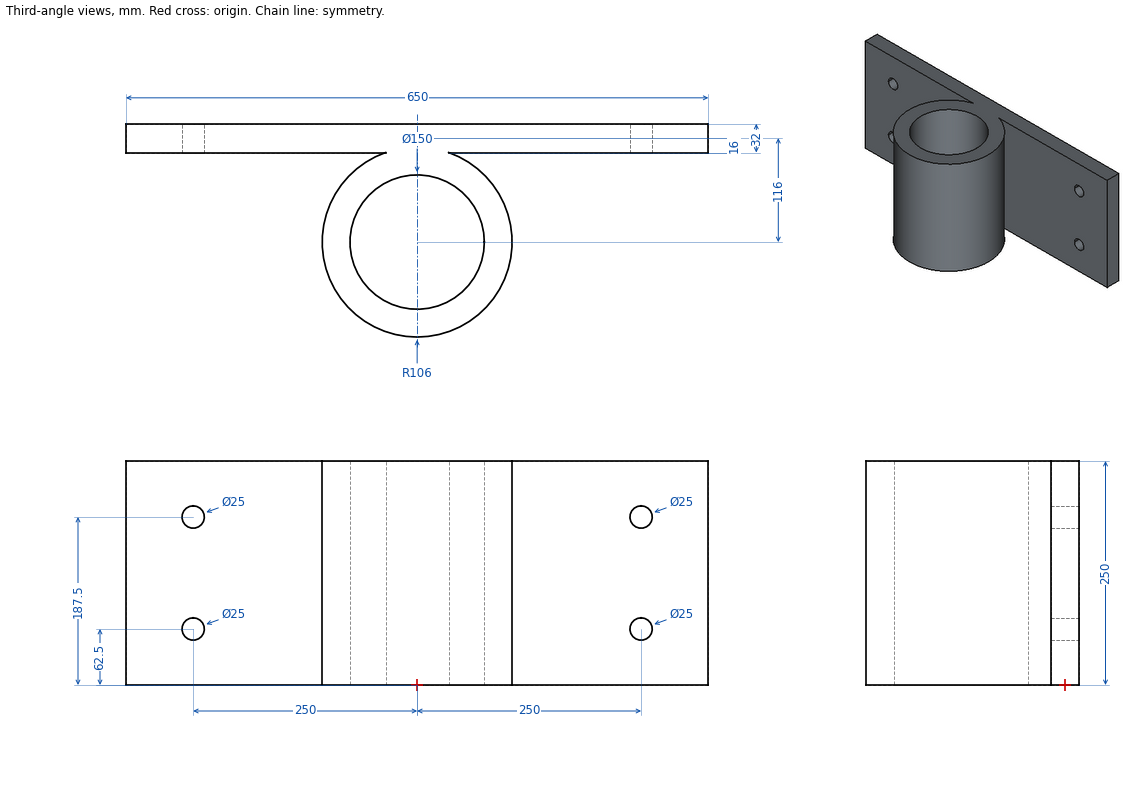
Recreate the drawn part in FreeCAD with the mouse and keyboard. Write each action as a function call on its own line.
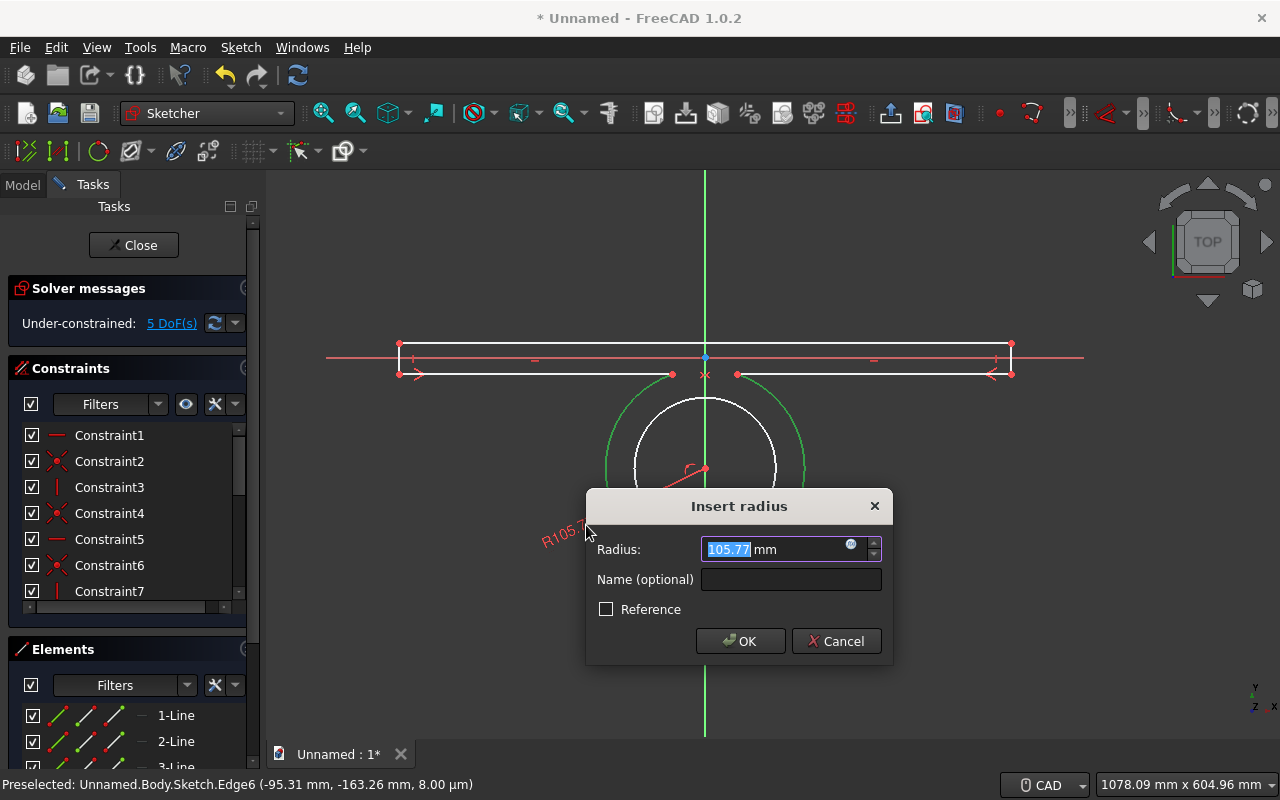
text(106)
key(Return)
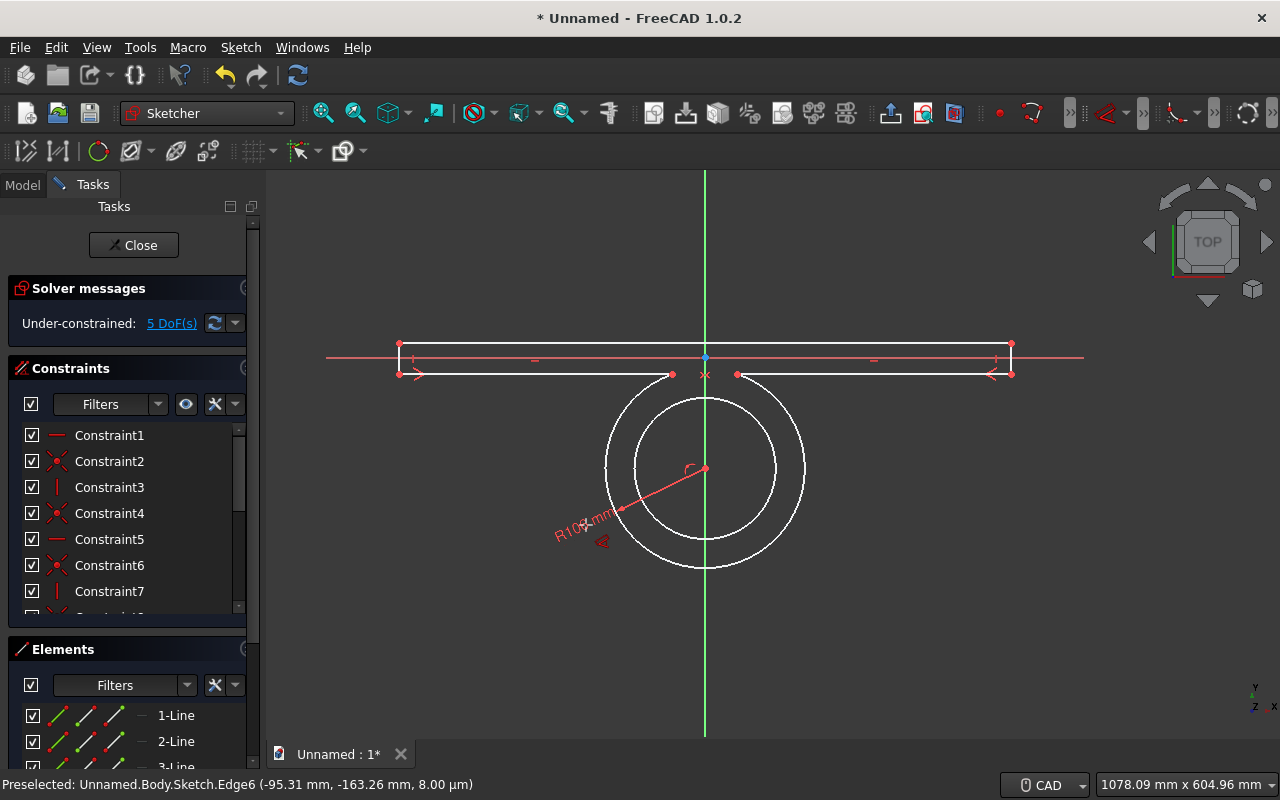
click(755, 418)
click(826, 432)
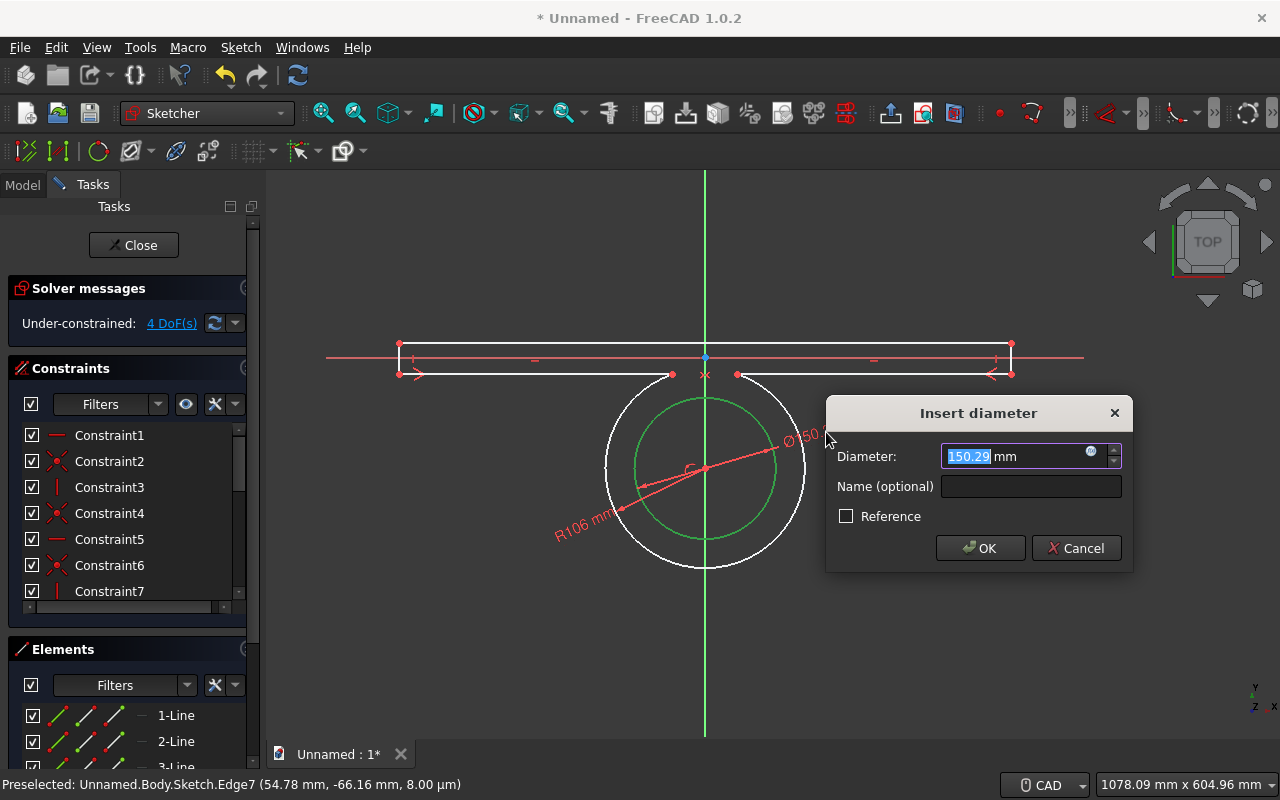
text(150)
key(Return)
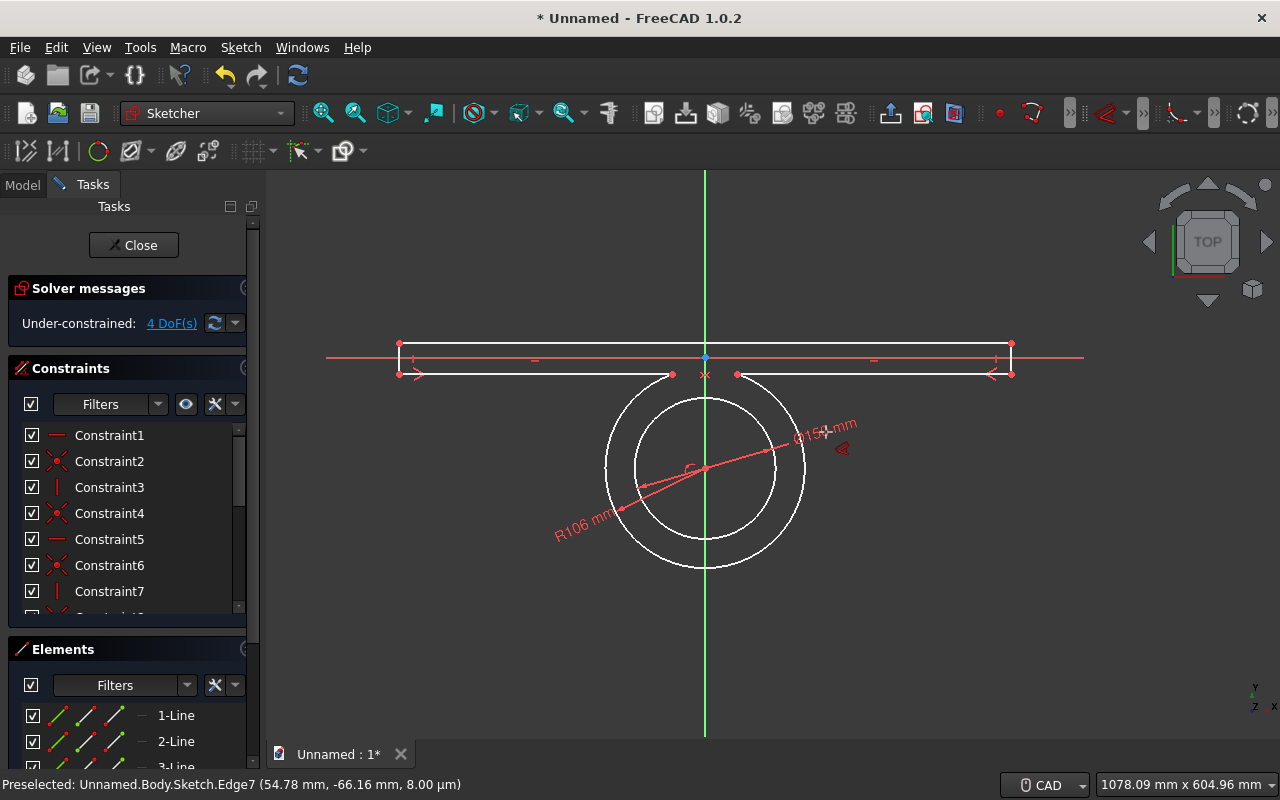
scroll(1011, 356, up, 2)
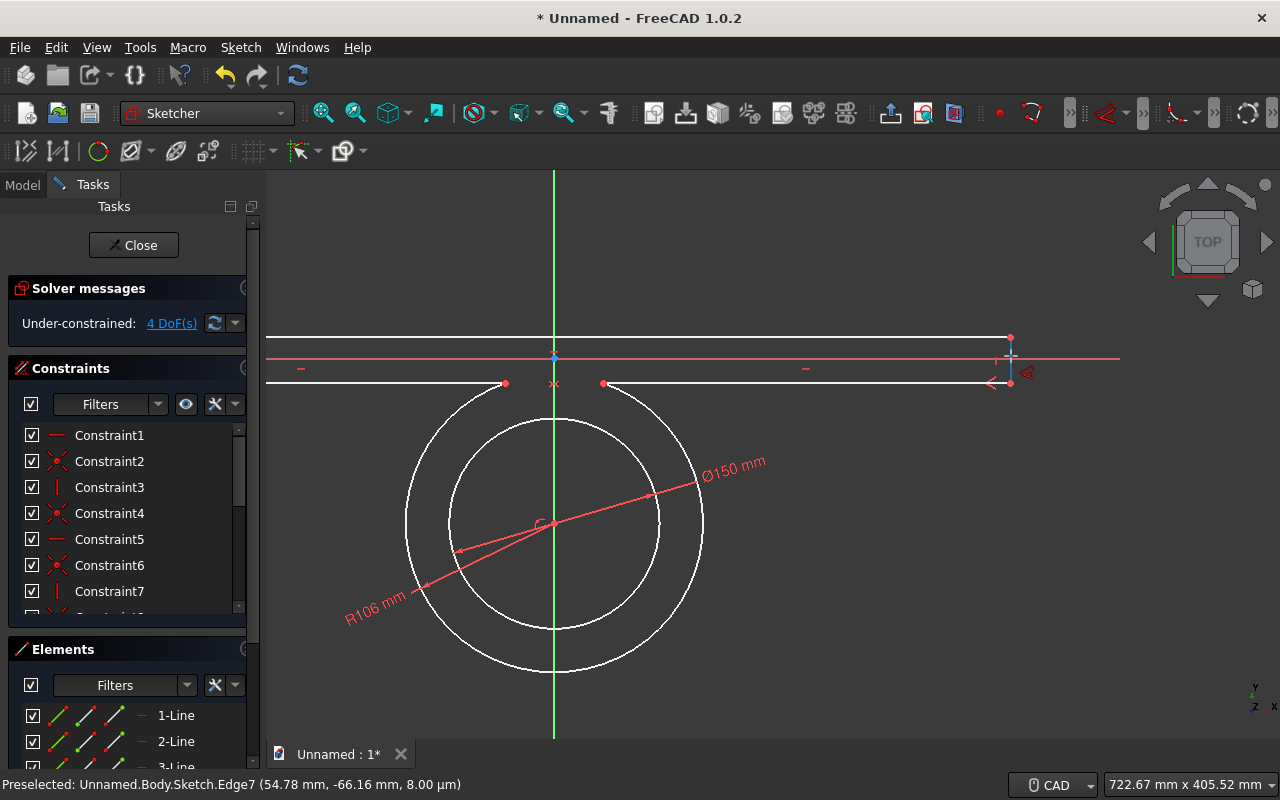
click(1011, 355)
click(1045, 344)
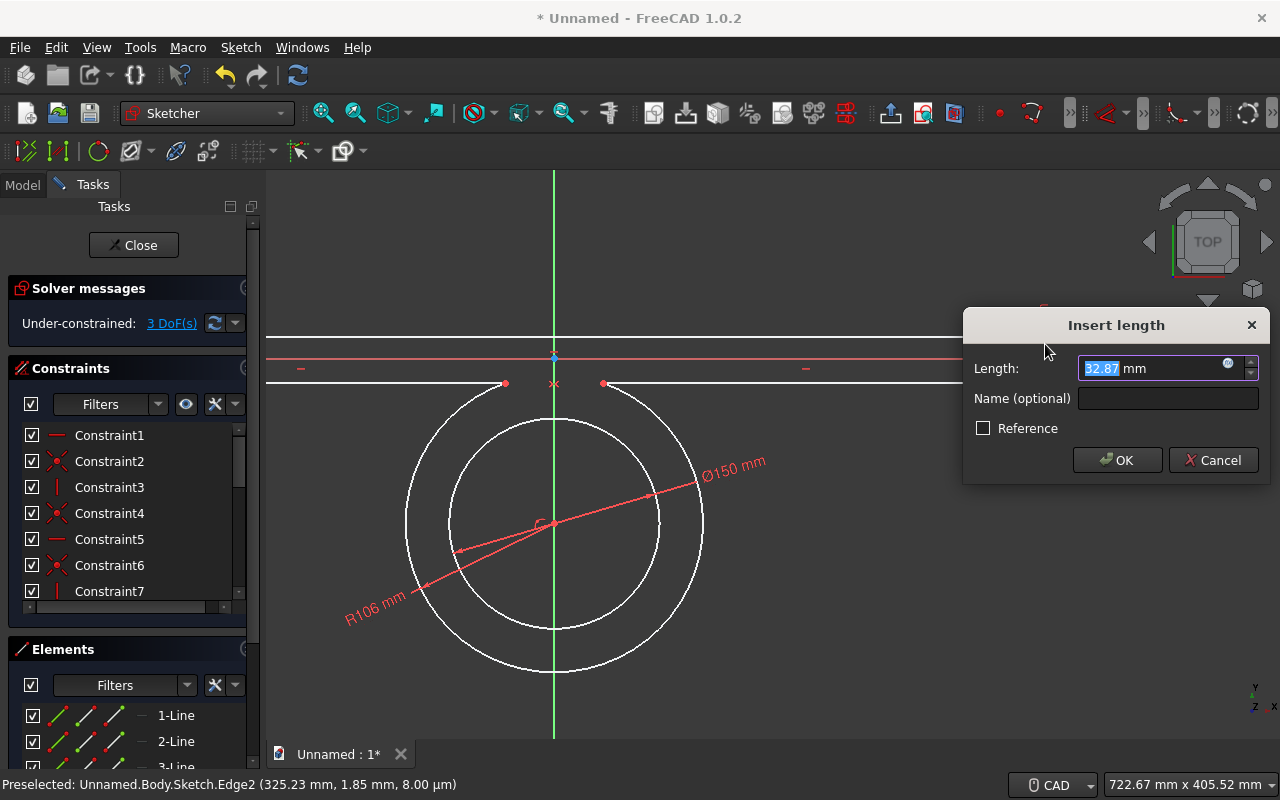
text(32)
key(Return)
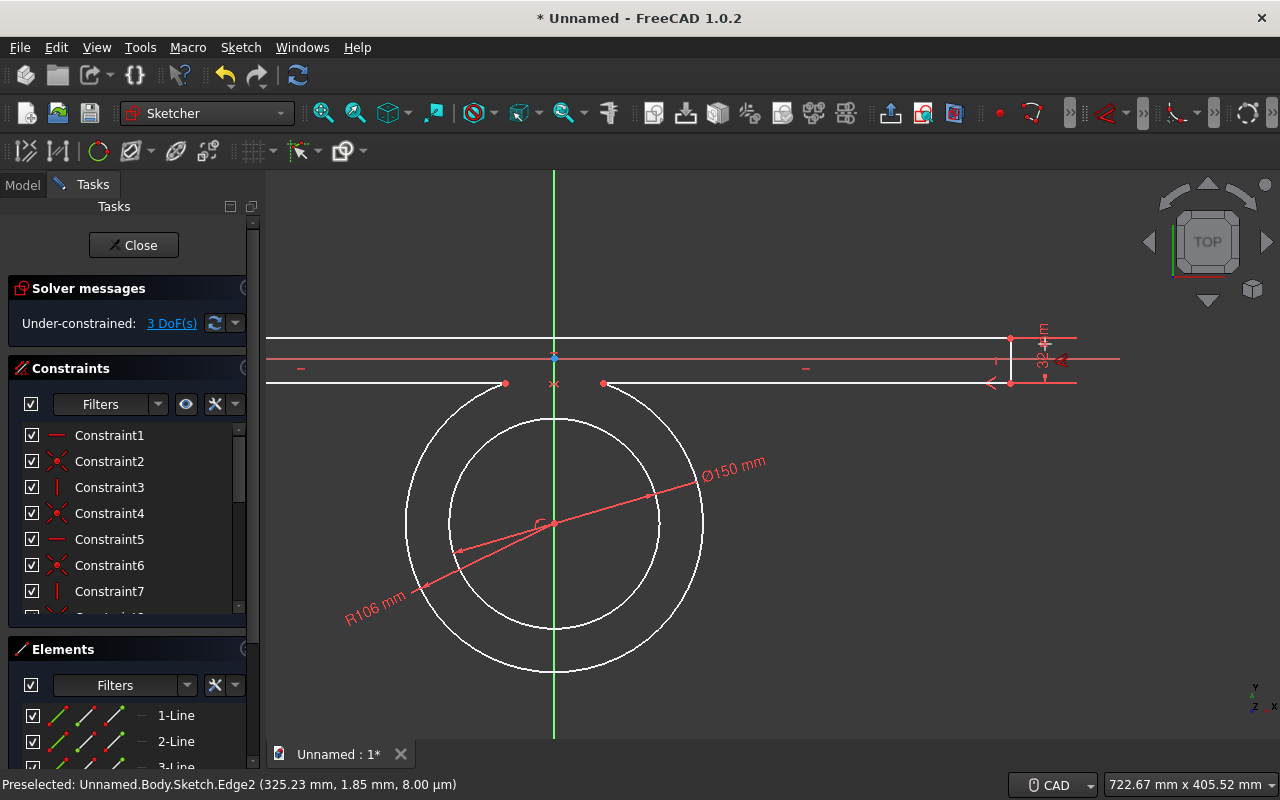
click(737, 338)
click(652, 304)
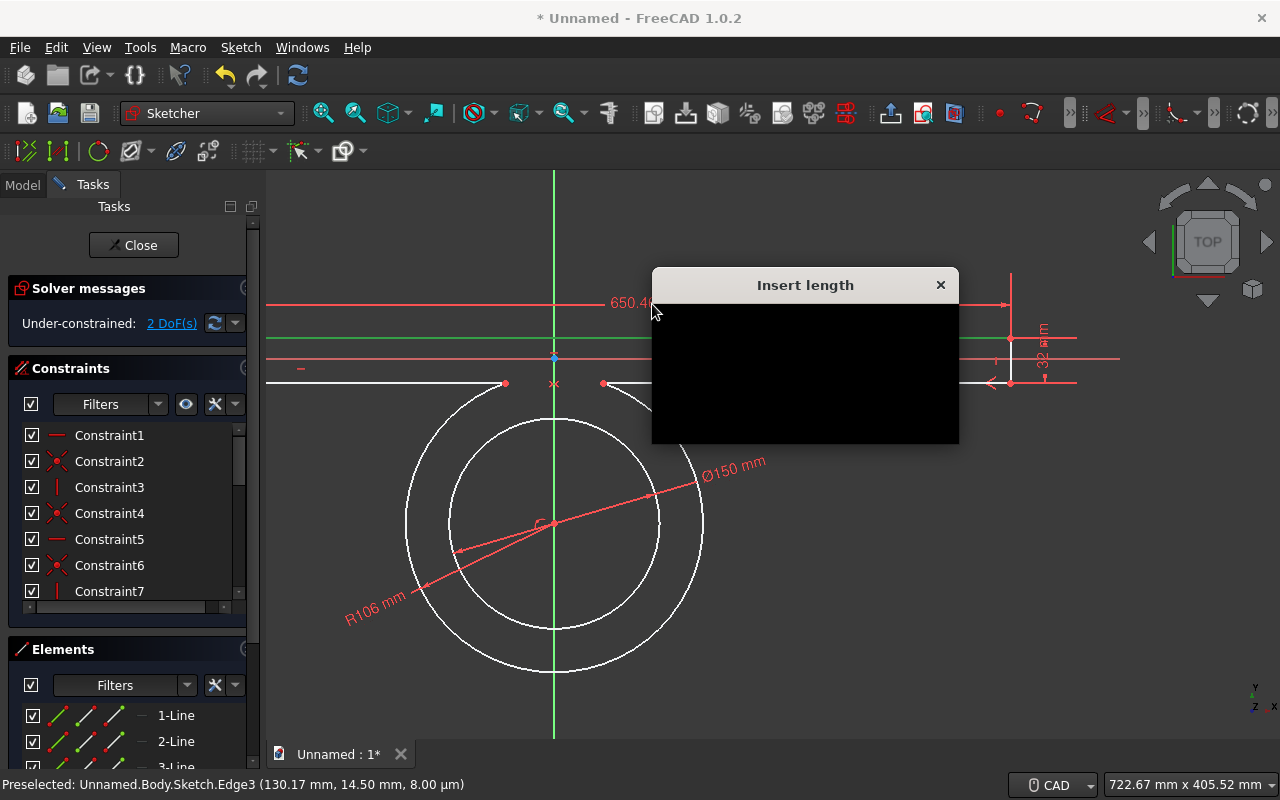
text(650)
key(Return)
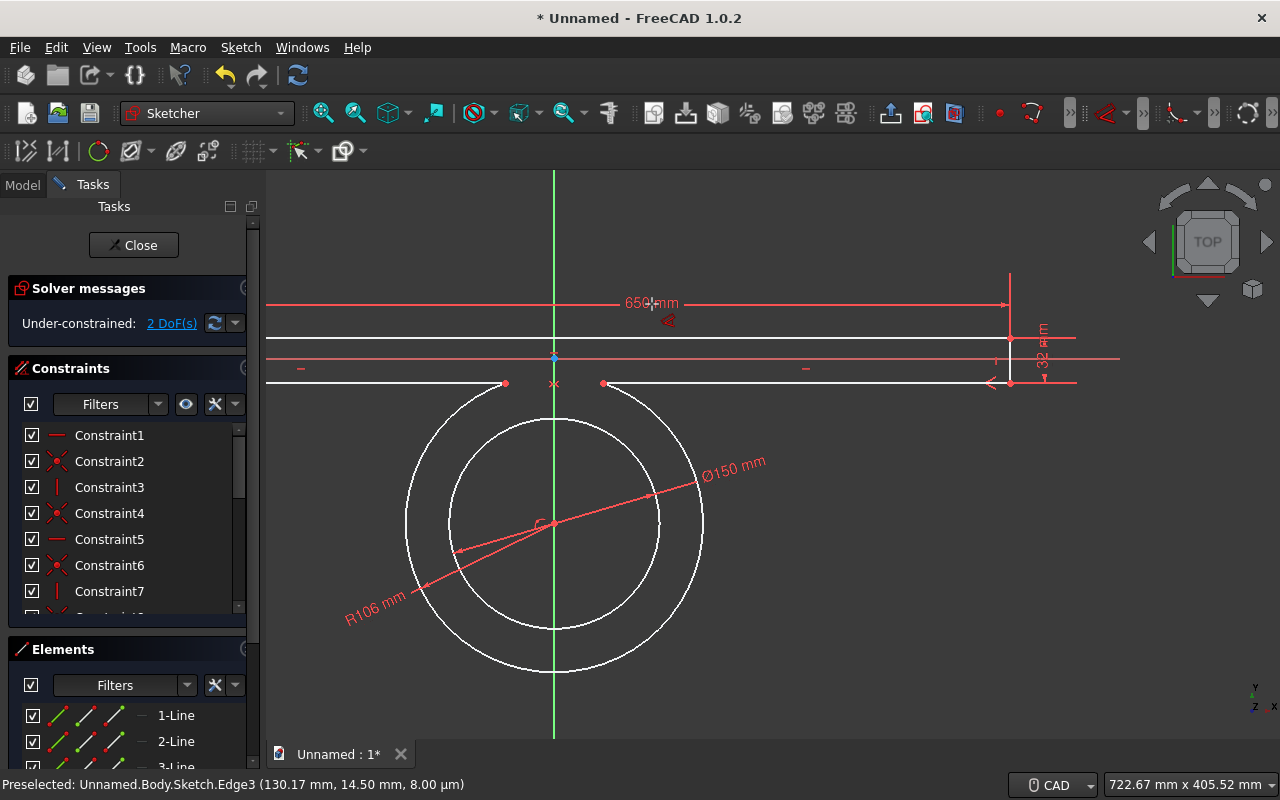
scroll(603, 383, up, 3)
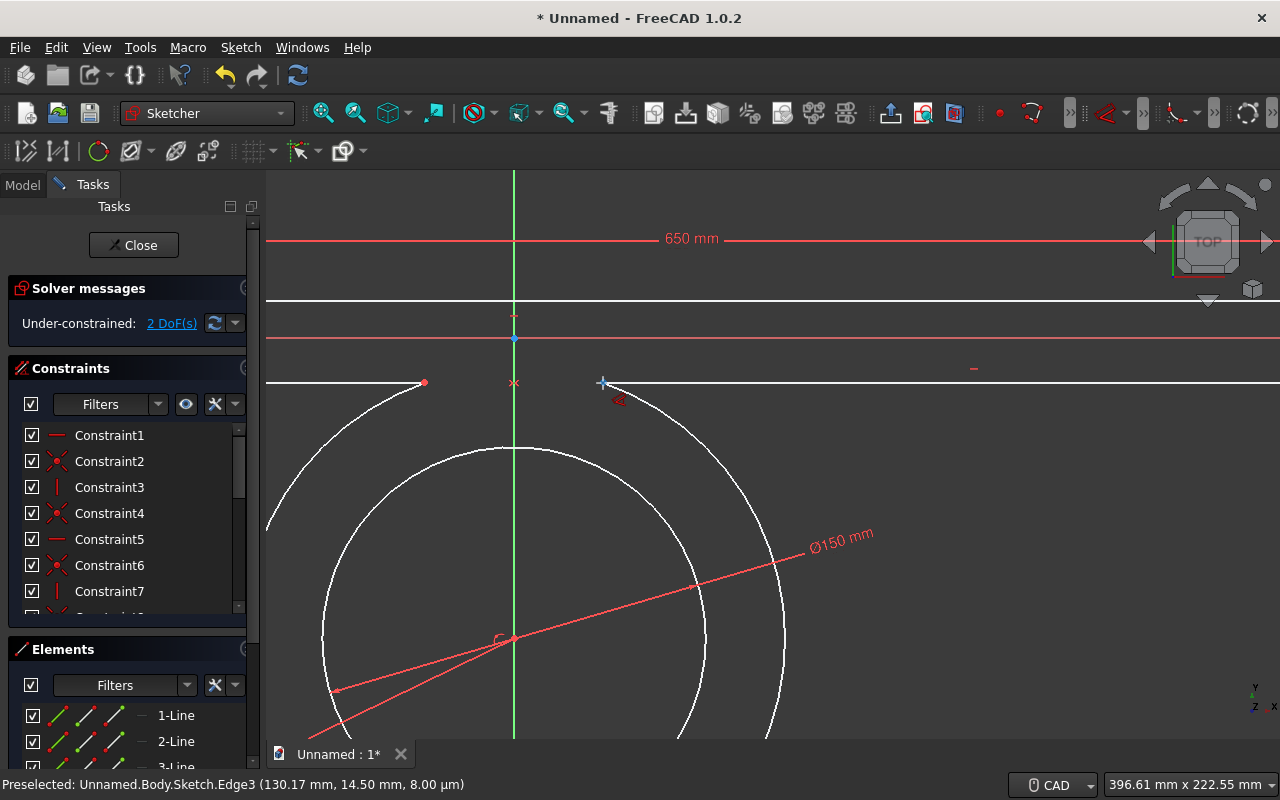
click(603, 383)
click(637, 361)